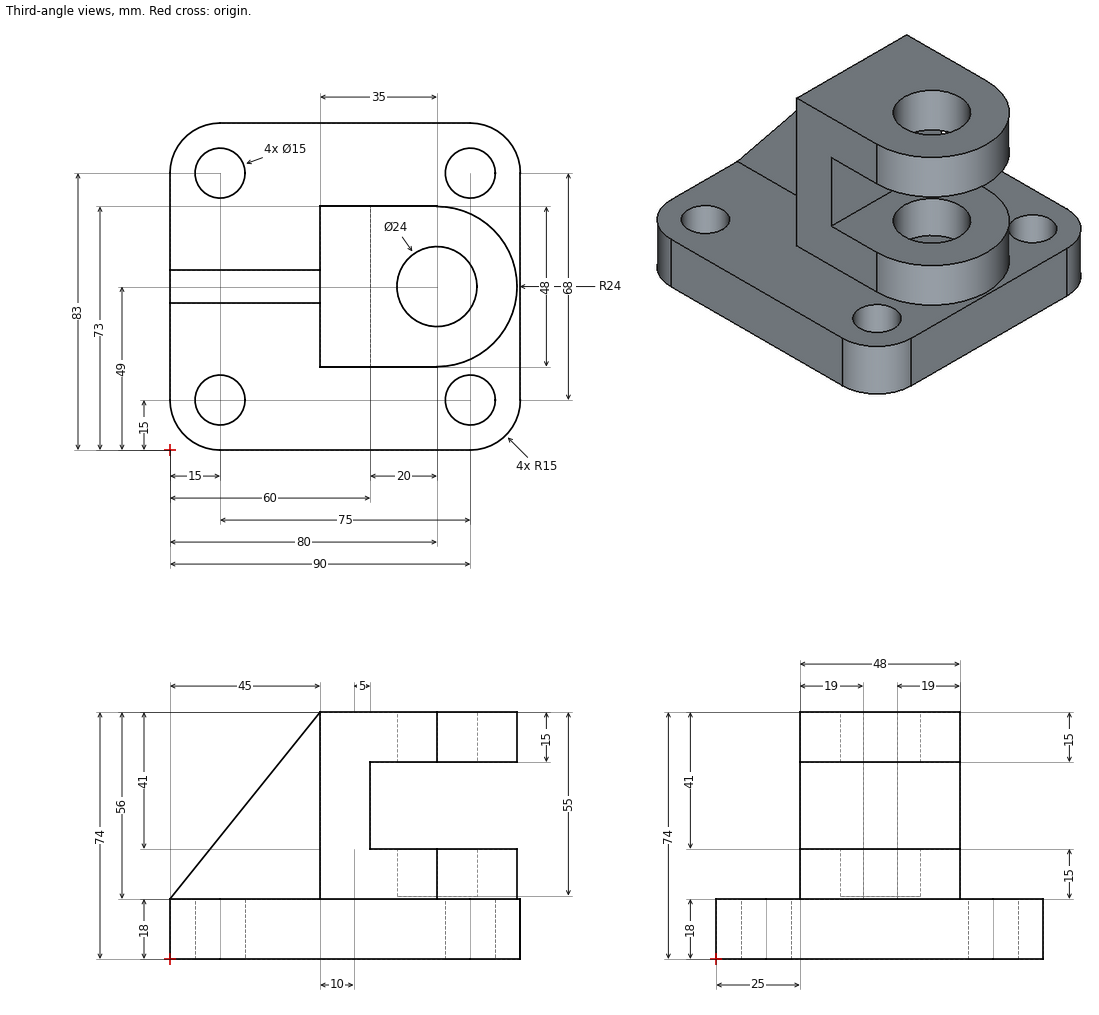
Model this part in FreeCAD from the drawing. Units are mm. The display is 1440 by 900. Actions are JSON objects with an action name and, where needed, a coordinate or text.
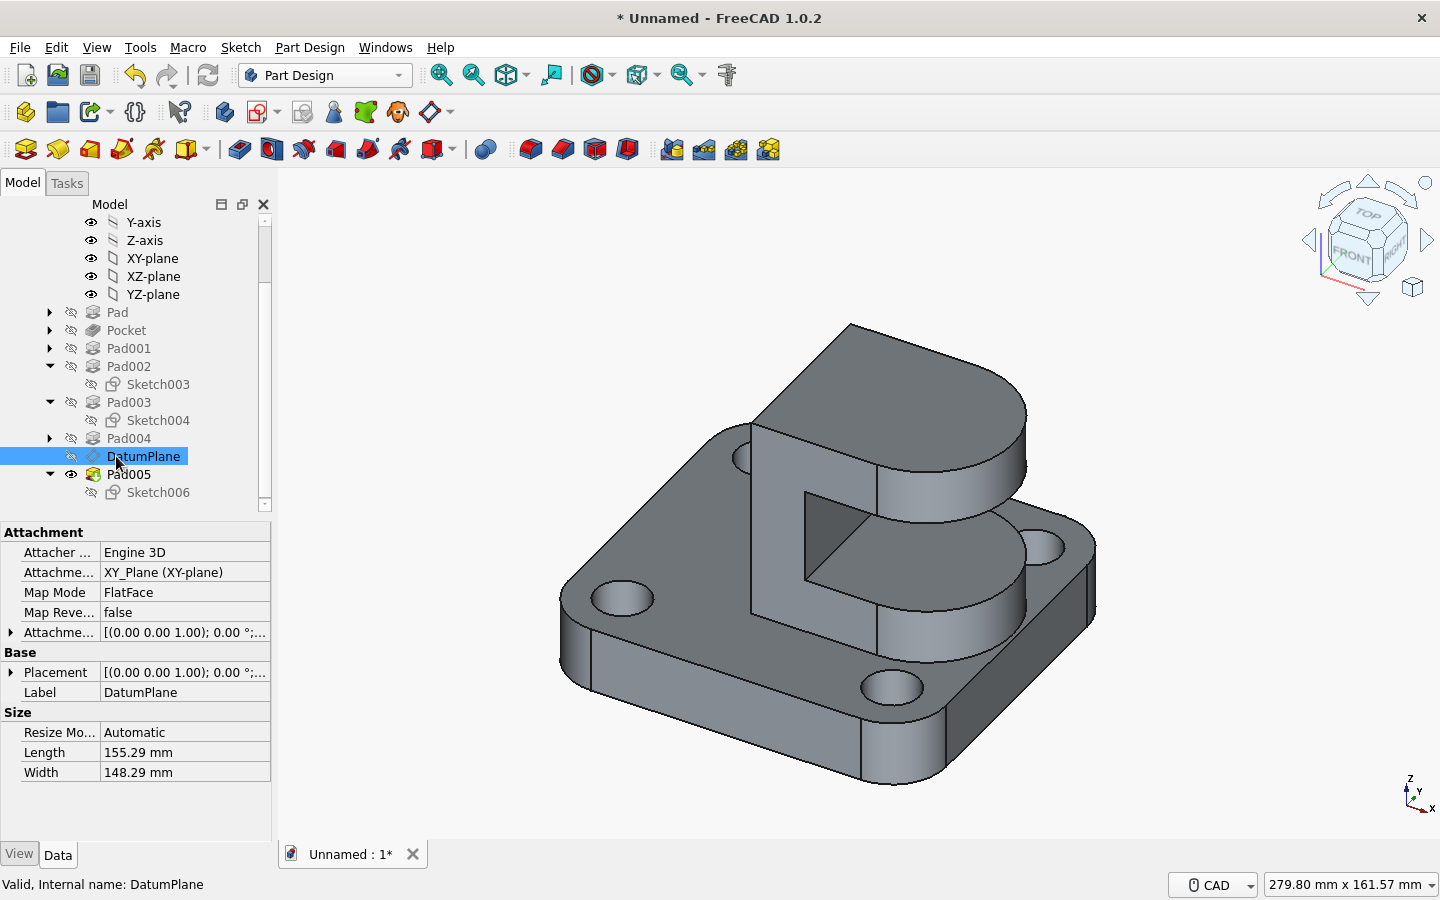
{"action": "left_click", "coordinate": [907, 408]}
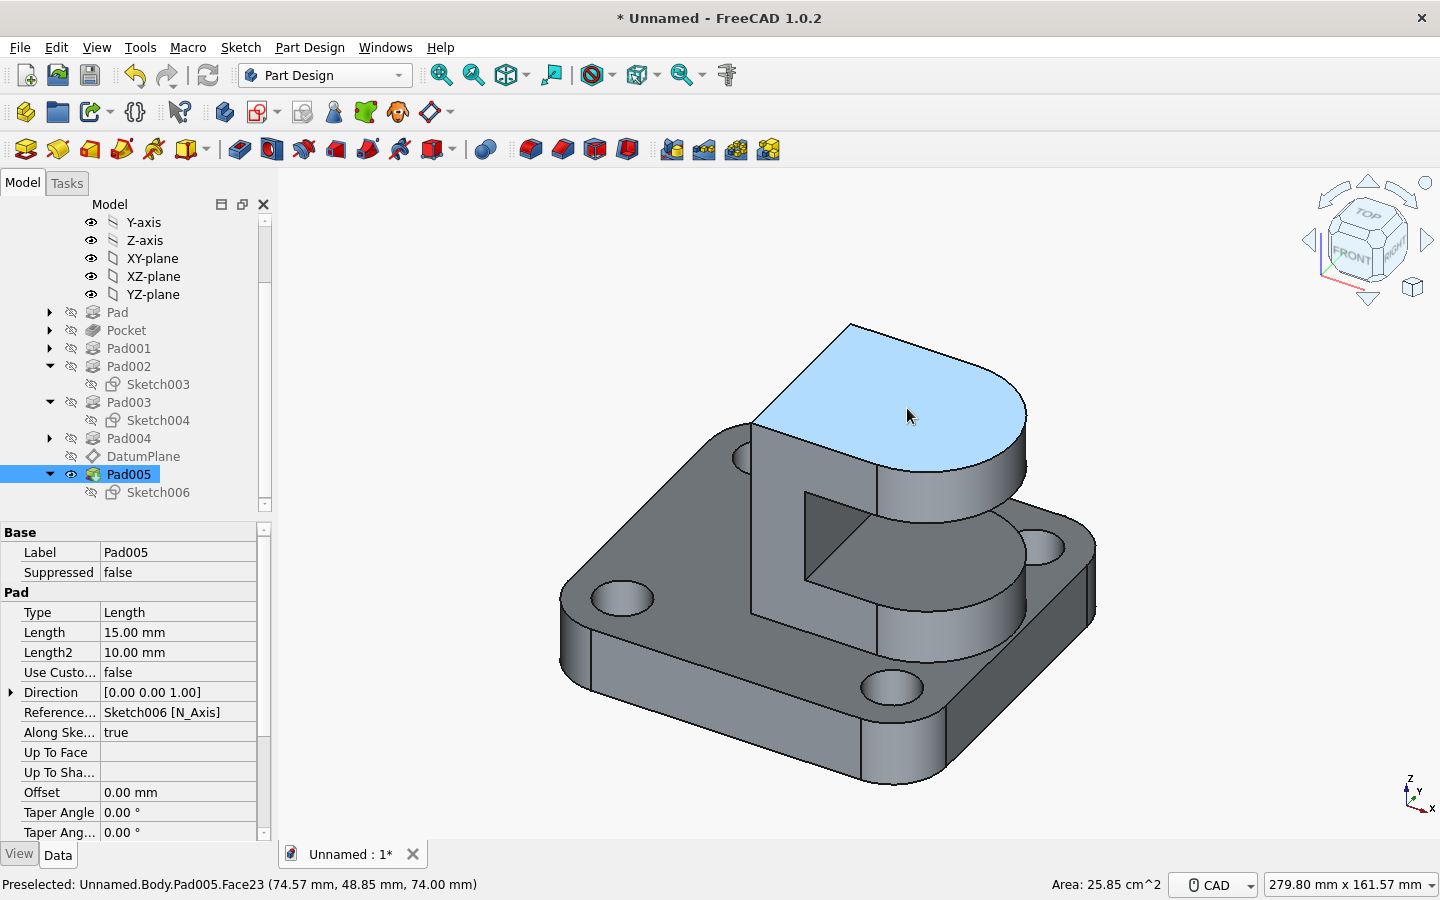
{"action": "left_click", "coordinate": [258, 112]}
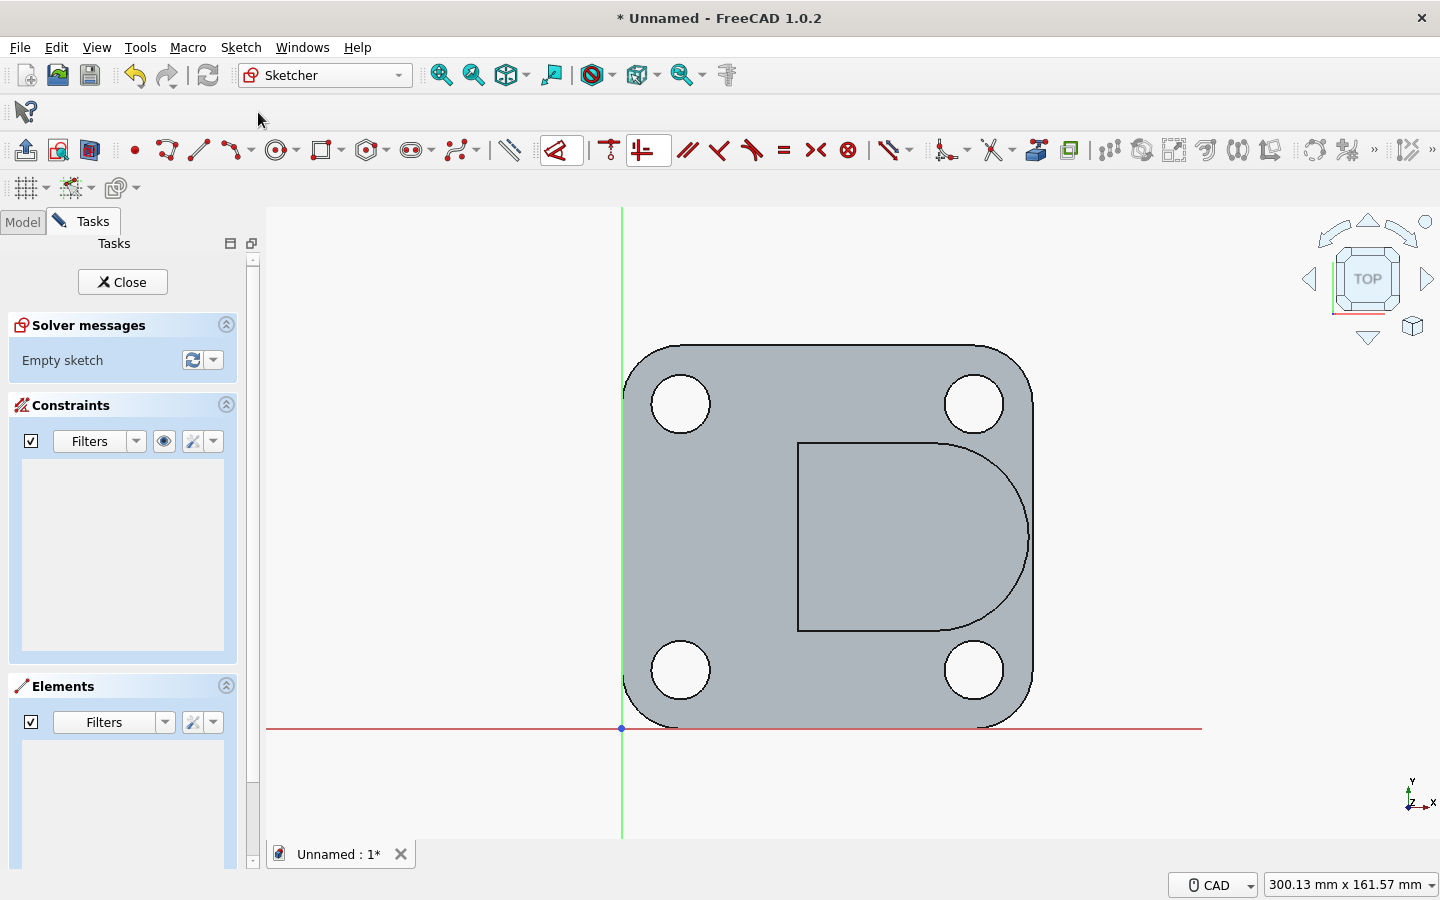
{"action": "scroll", "coordinate": [984, 542], "scroll_direction": "up", "scroll_amount": 7}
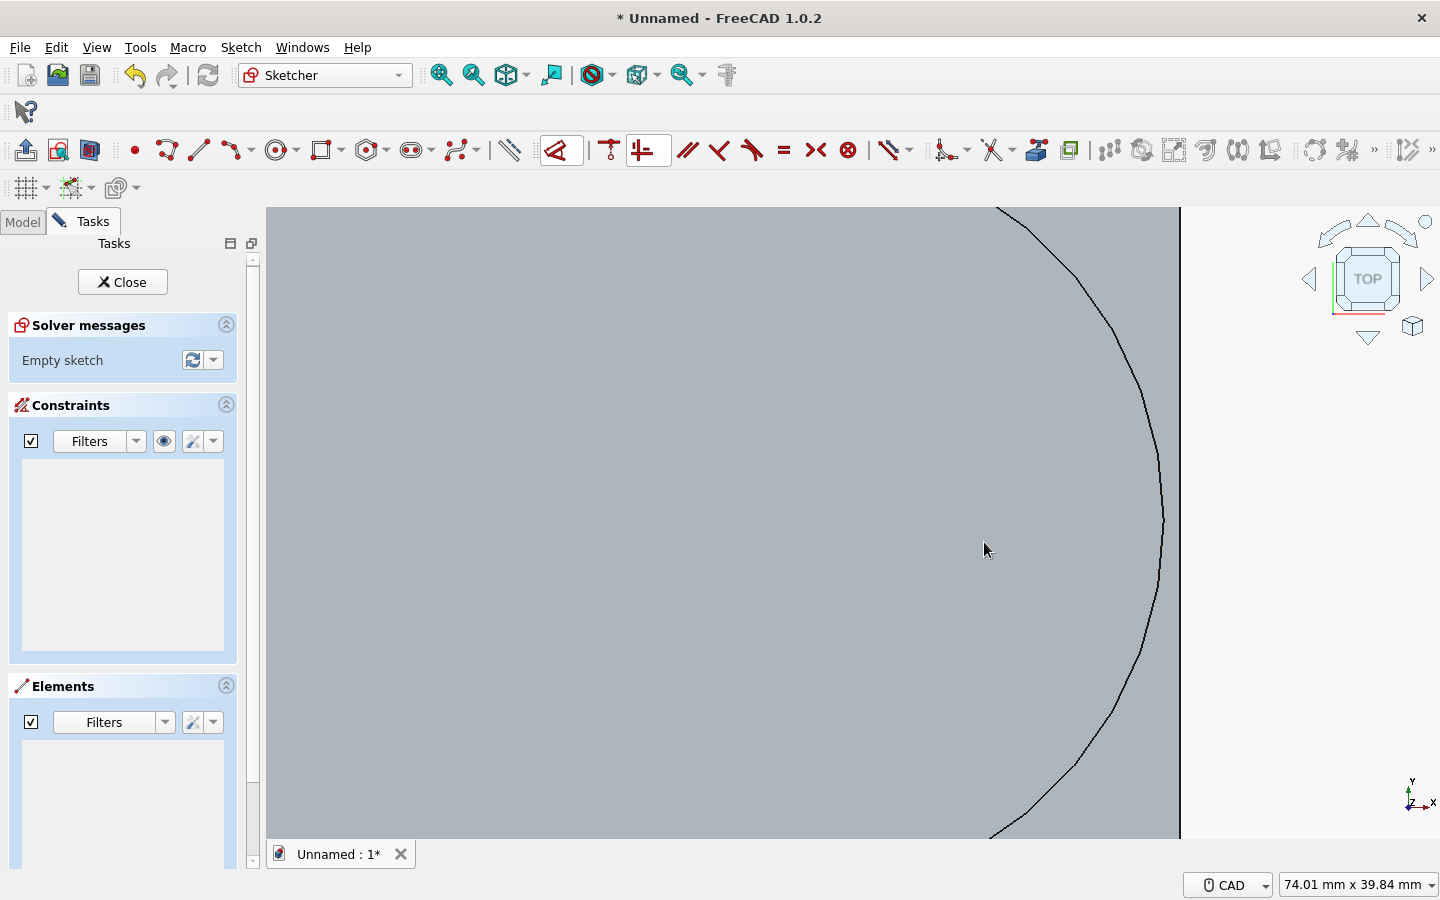
{"action": "left_click", "coordinate": [276, 150]}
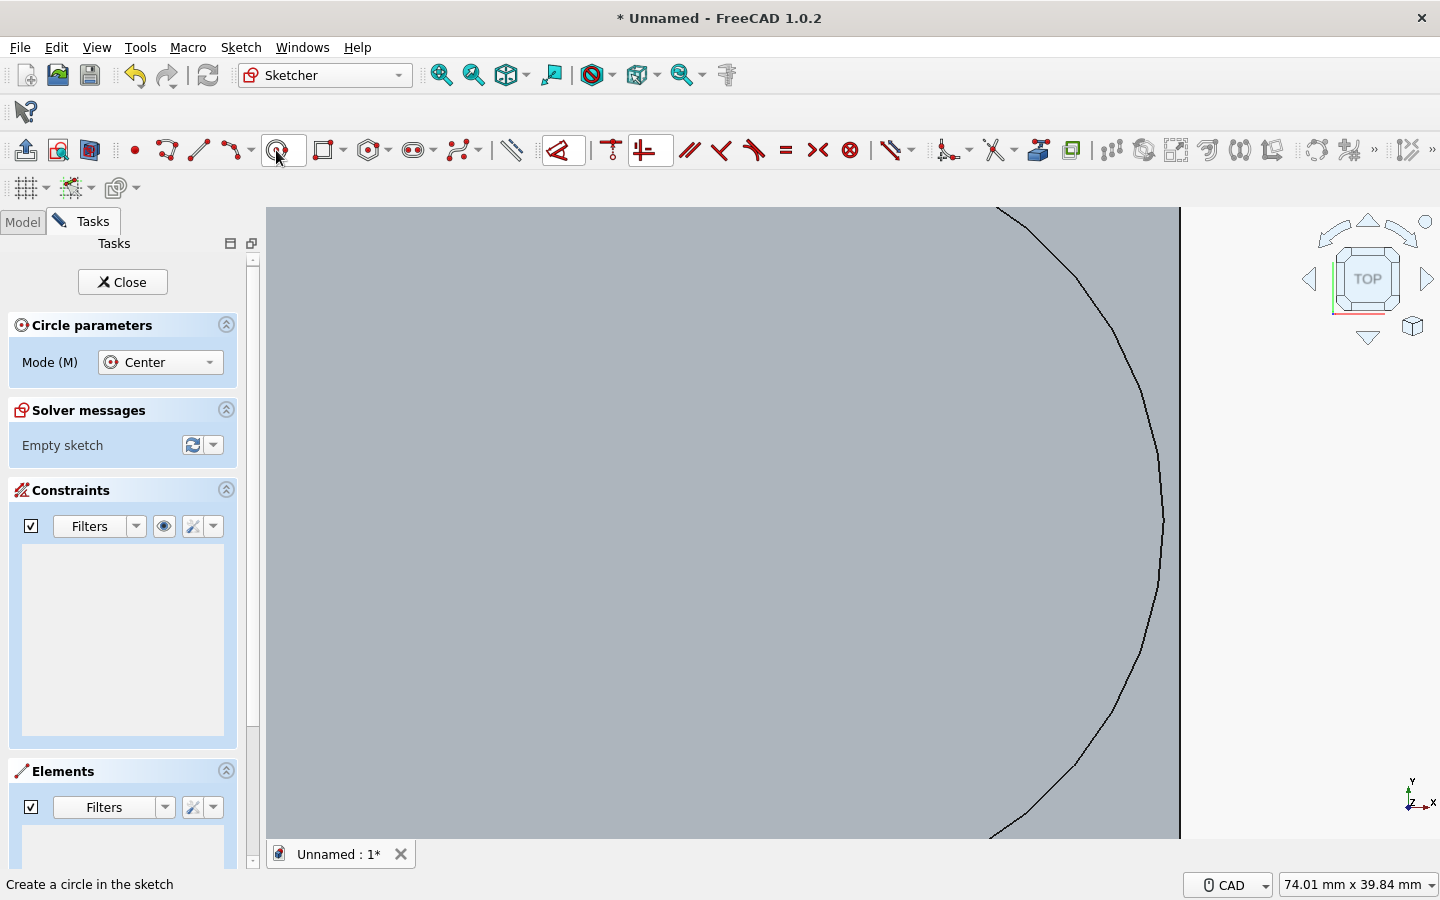
{"action": "left_click", "coordinate": [783, 521]}
{"action": "left_click", "coordinate": [918, 386]}
{"action": "key", "text": "Escape"}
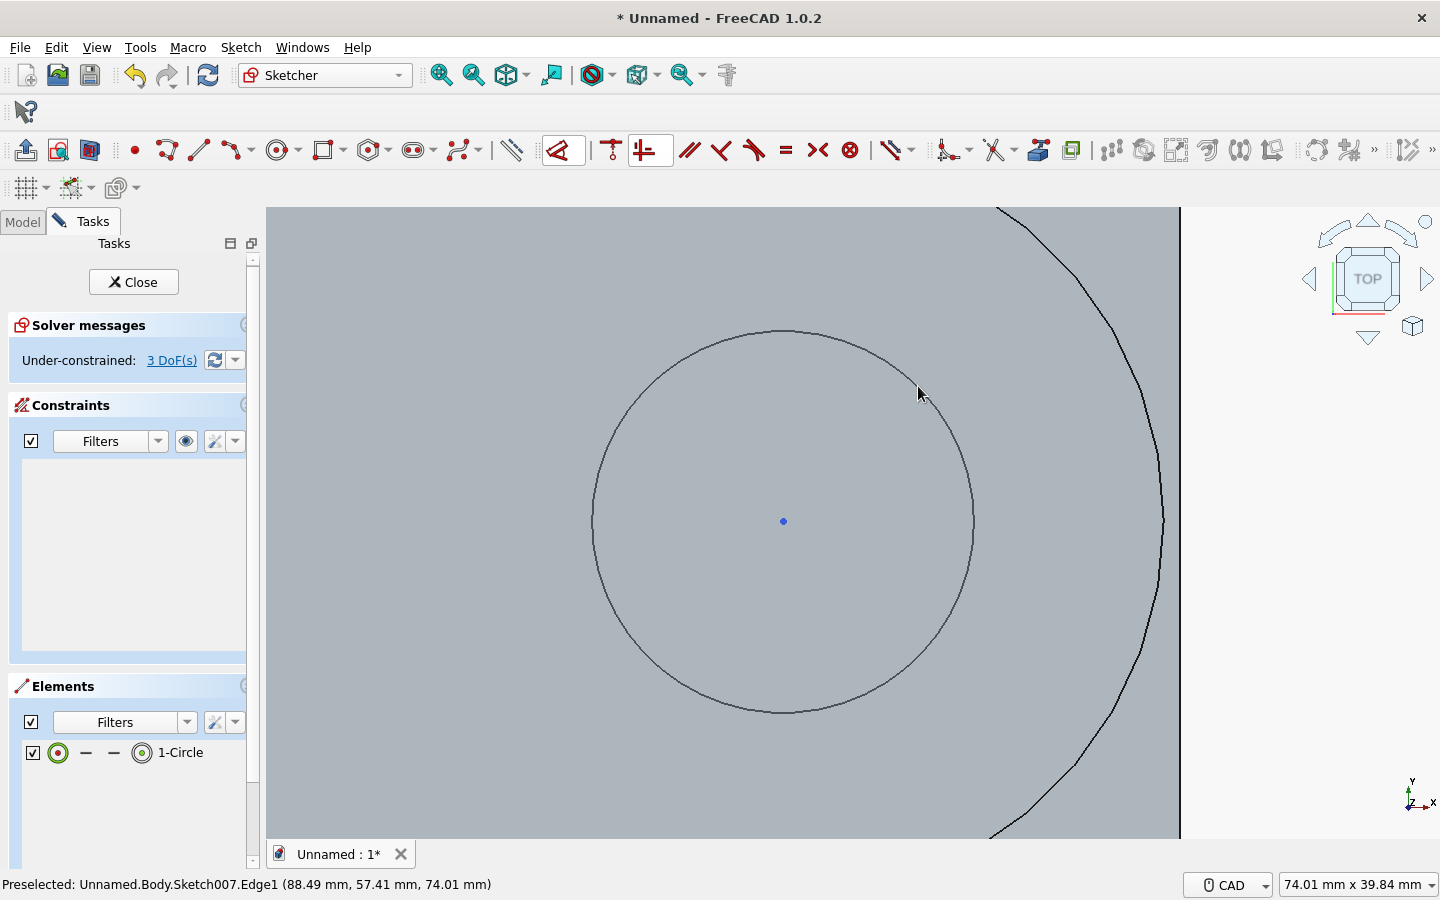
{"action": "left_click", "coordinate": [918, 387]}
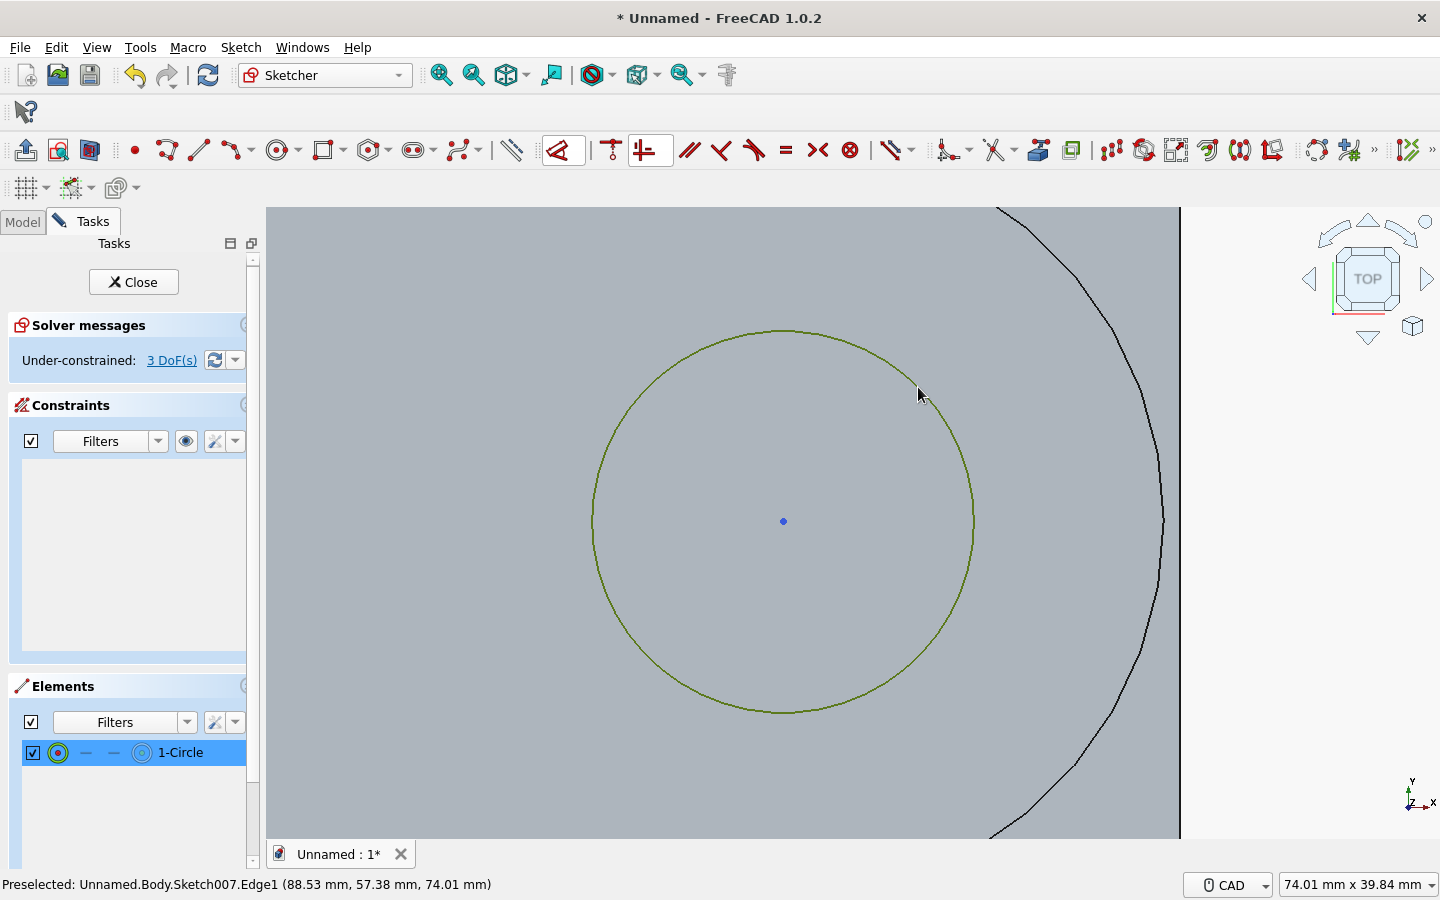
{"action": "left_click", "coordinate": [580, 150]}